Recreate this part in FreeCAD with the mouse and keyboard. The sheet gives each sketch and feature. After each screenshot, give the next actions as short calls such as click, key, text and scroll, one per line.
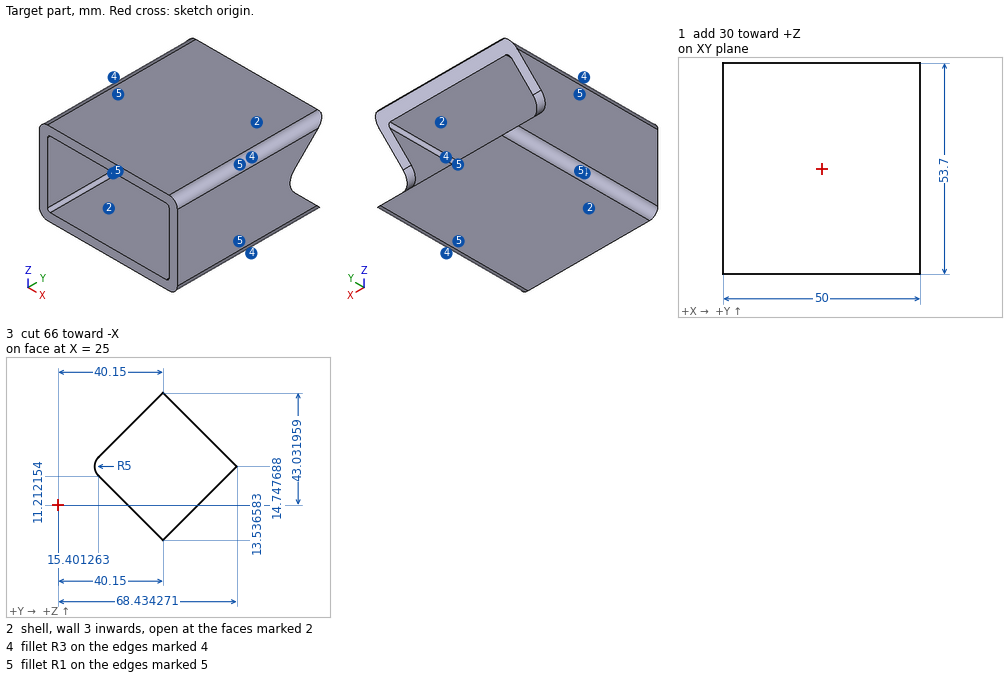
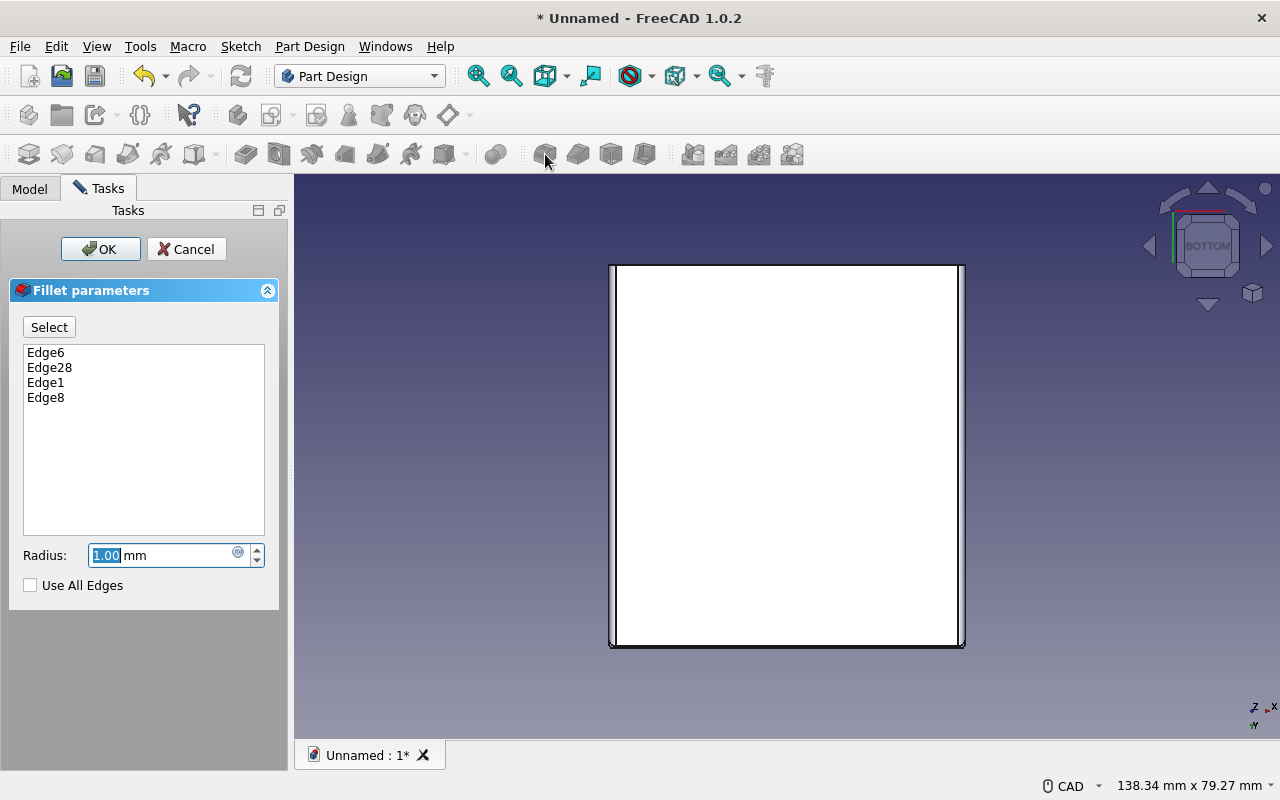
text(3)
key(Tab)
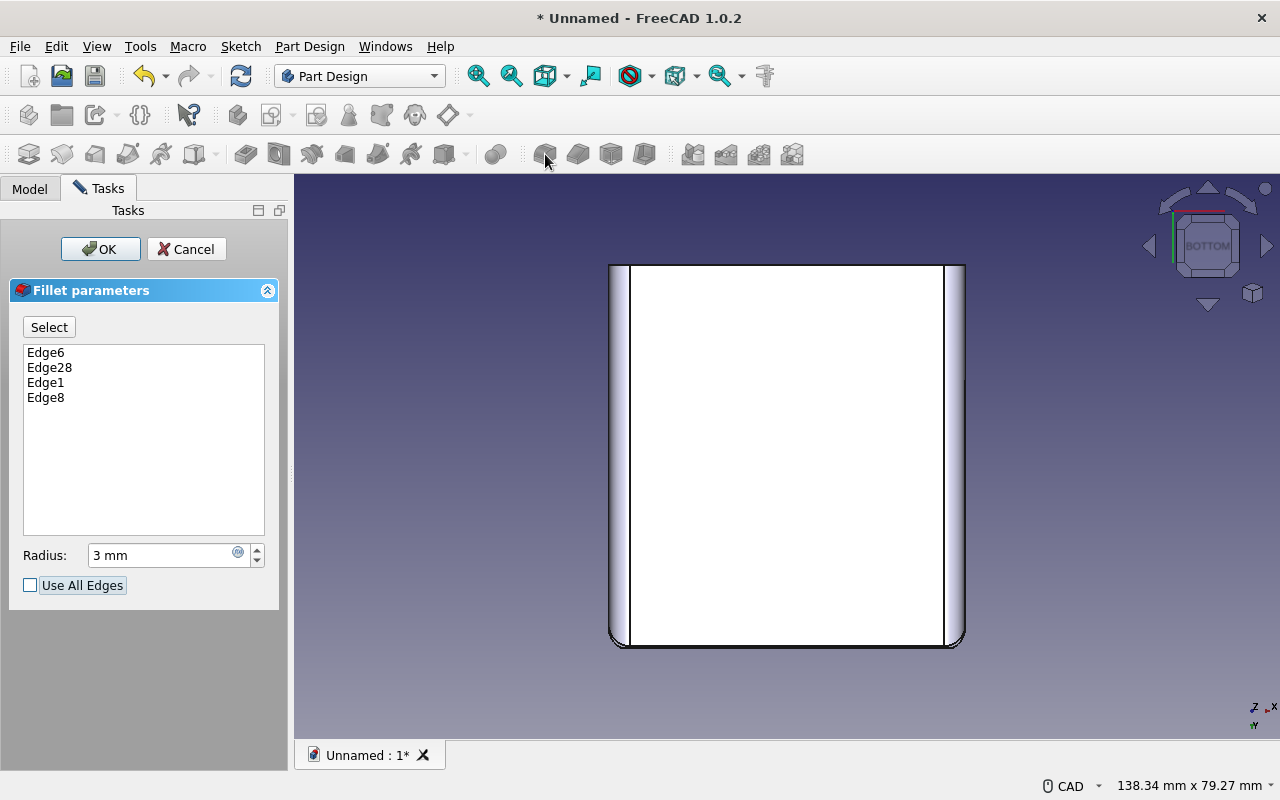
click(101, 249)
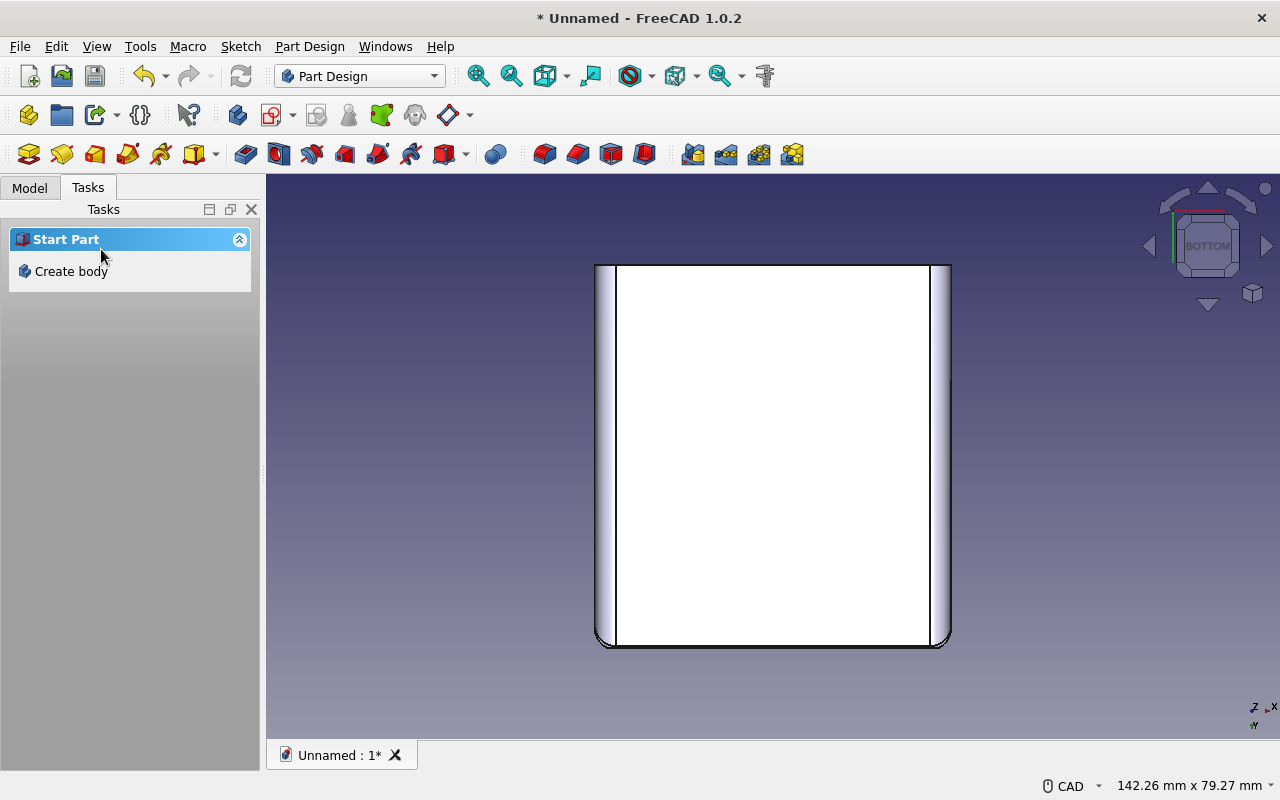
key(0)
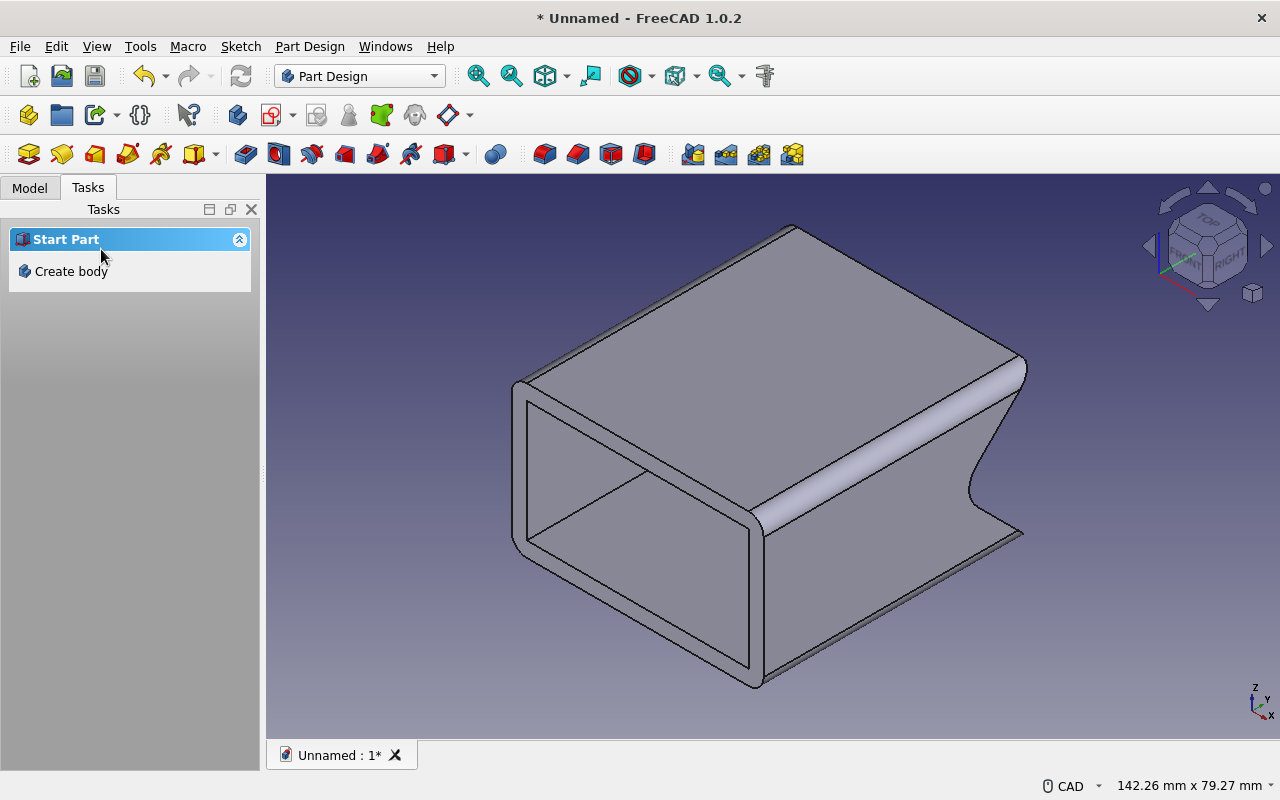
key(2)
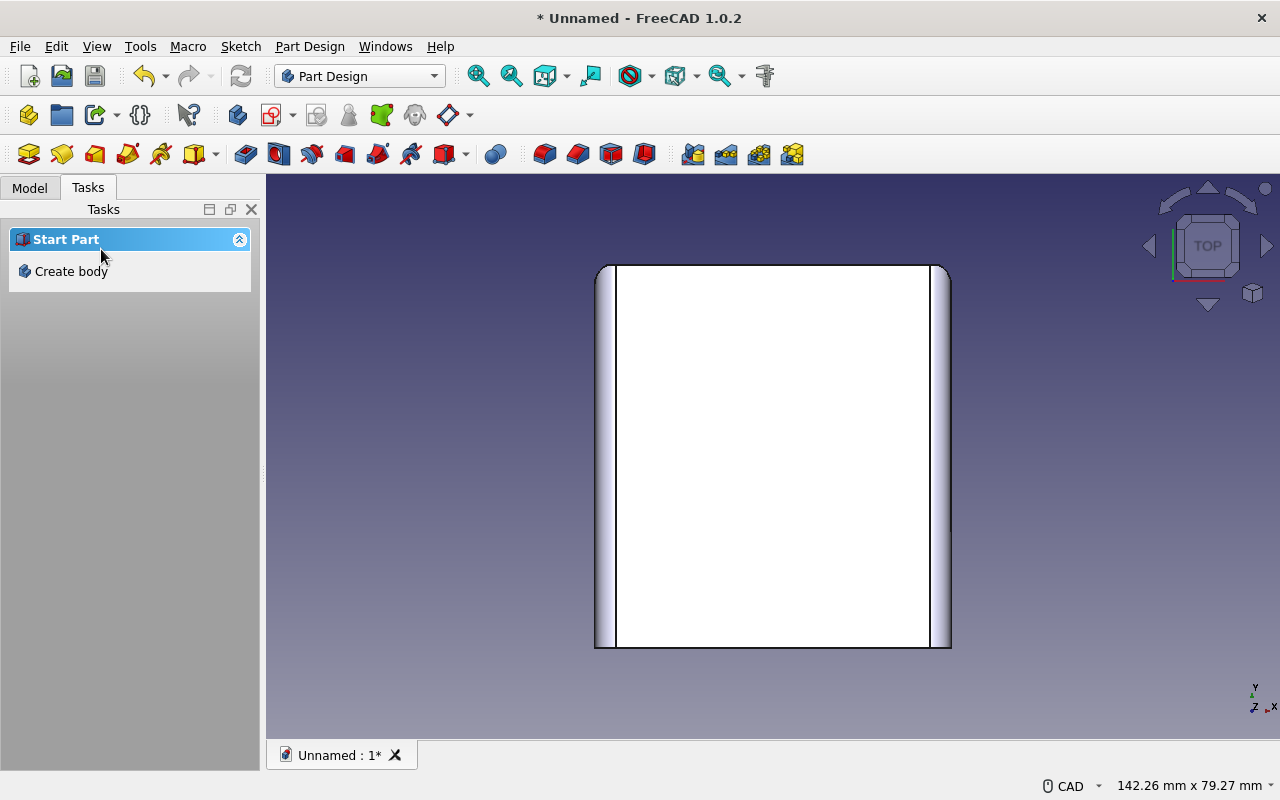
key(1)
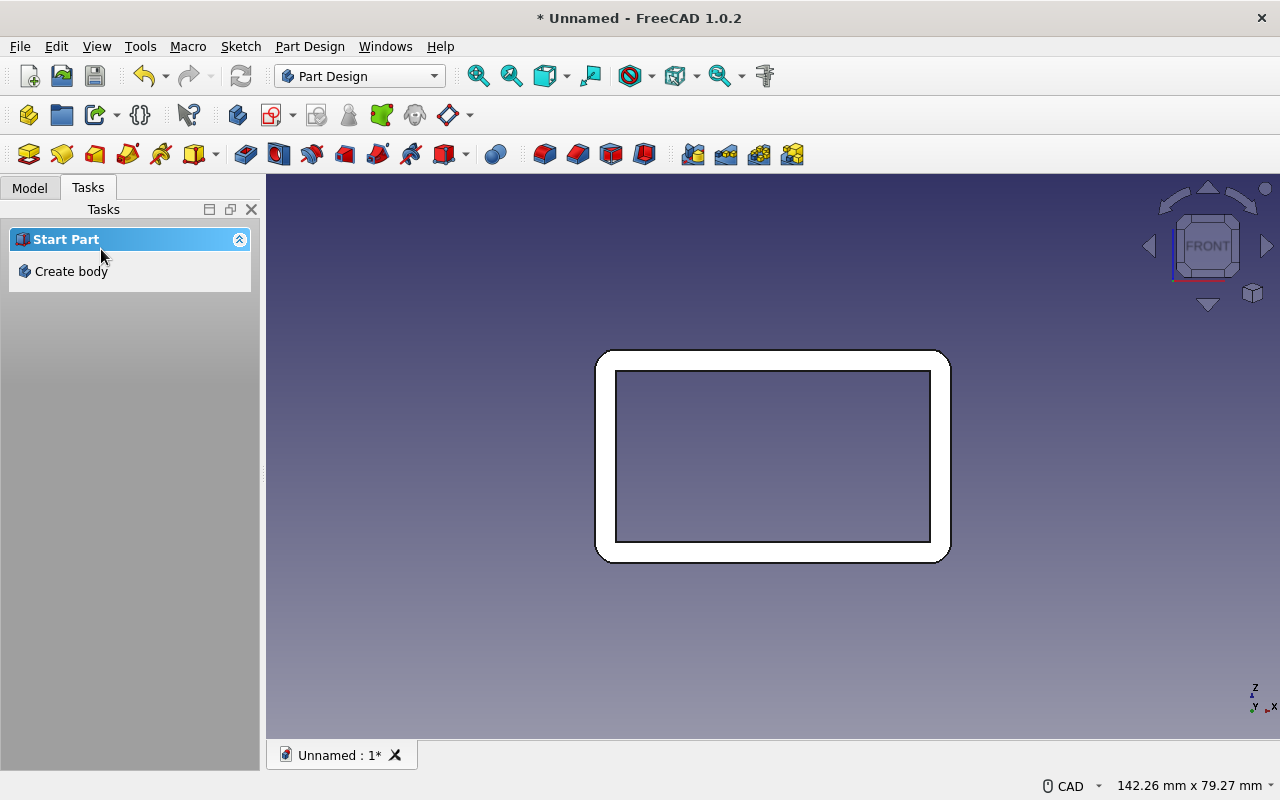
key(v)
key(f)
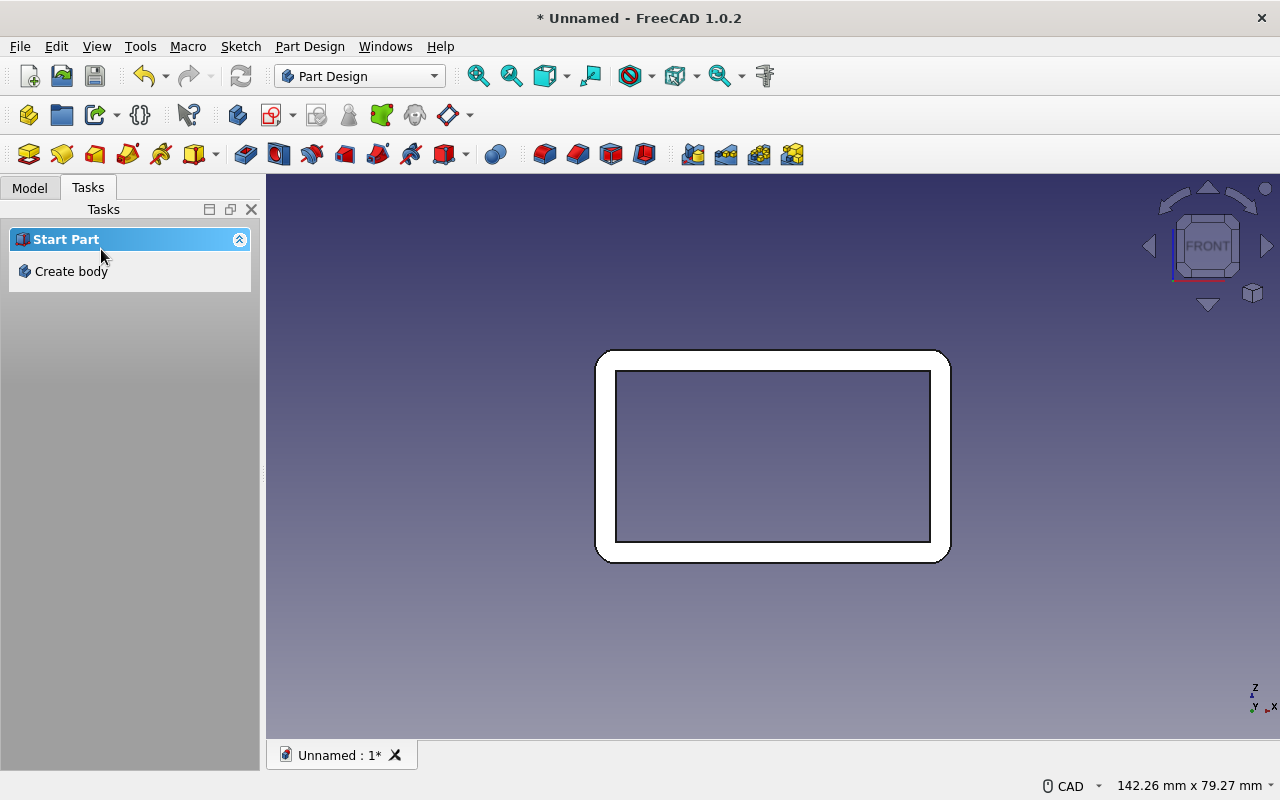
key(3)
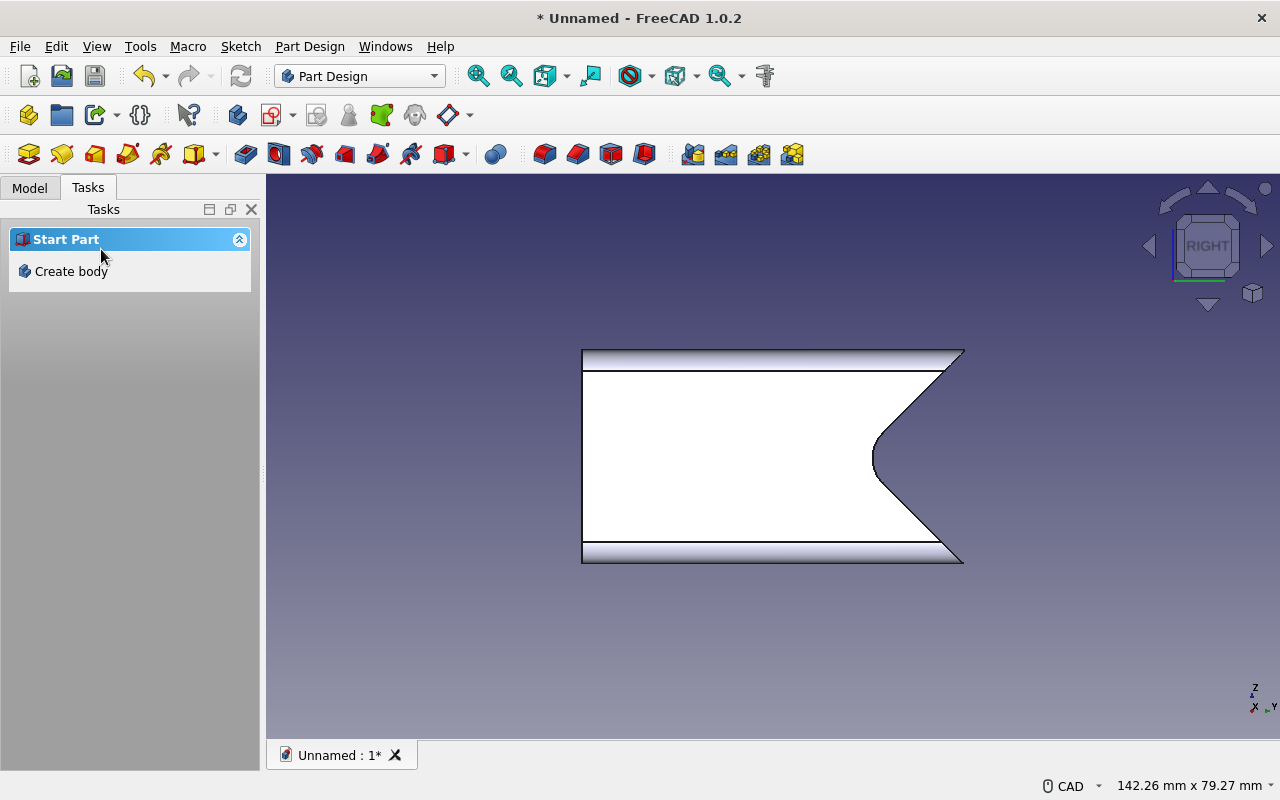
key(v)
key(f)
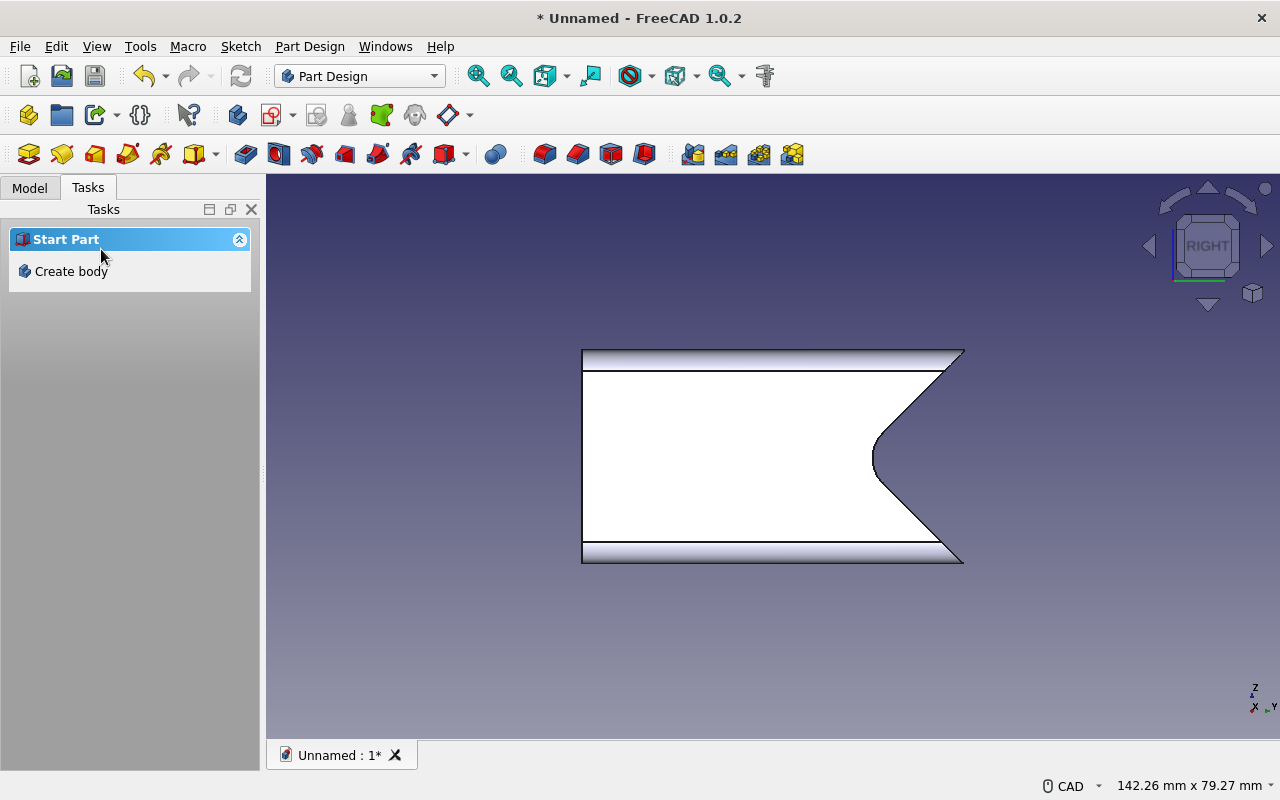
key(5)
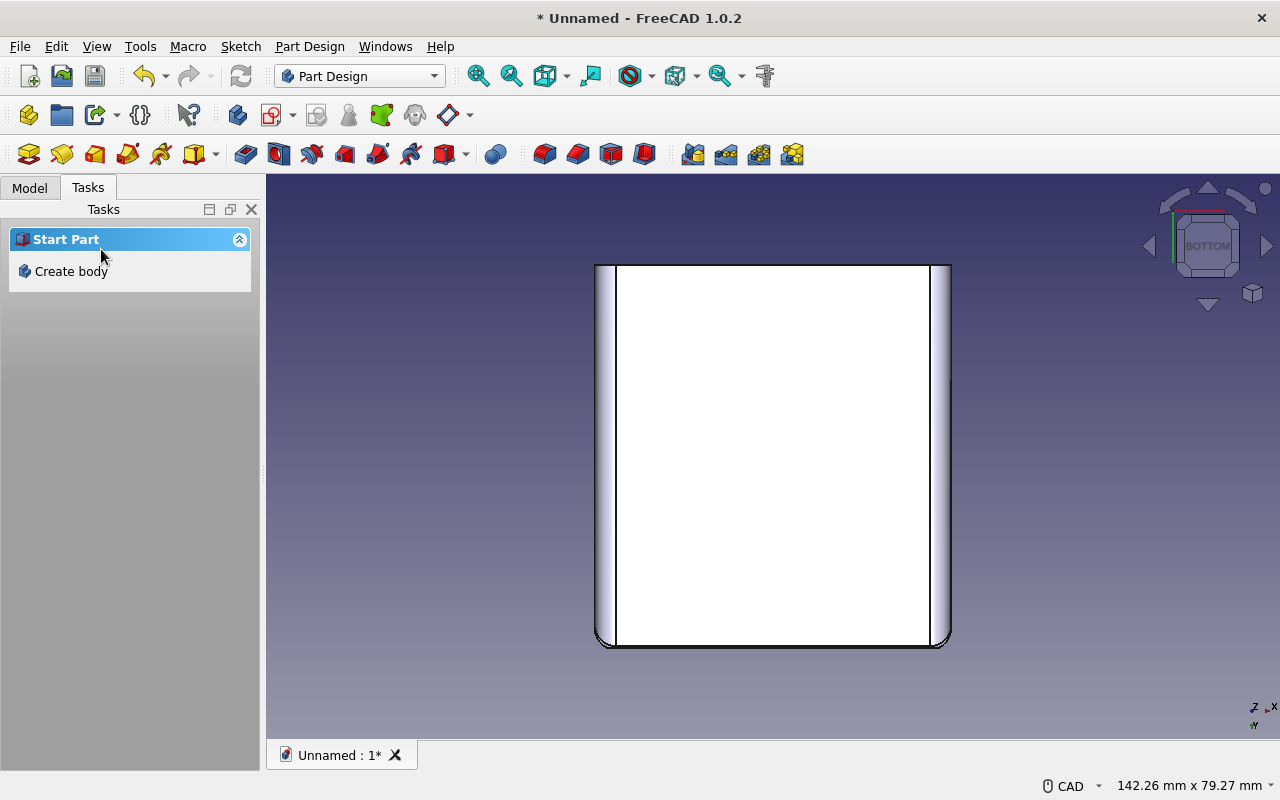
key(4)